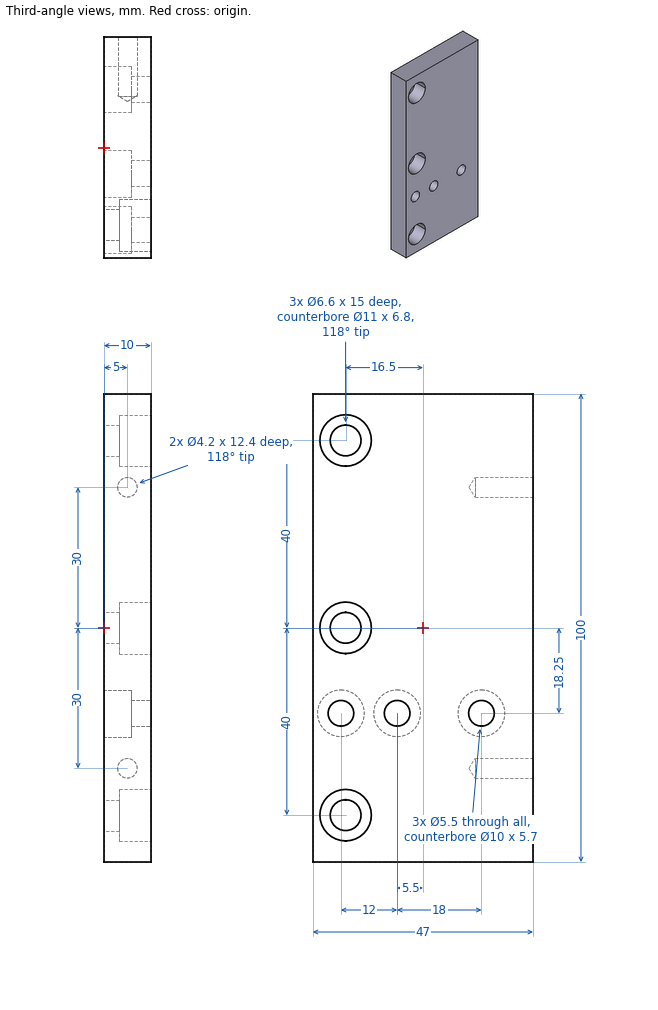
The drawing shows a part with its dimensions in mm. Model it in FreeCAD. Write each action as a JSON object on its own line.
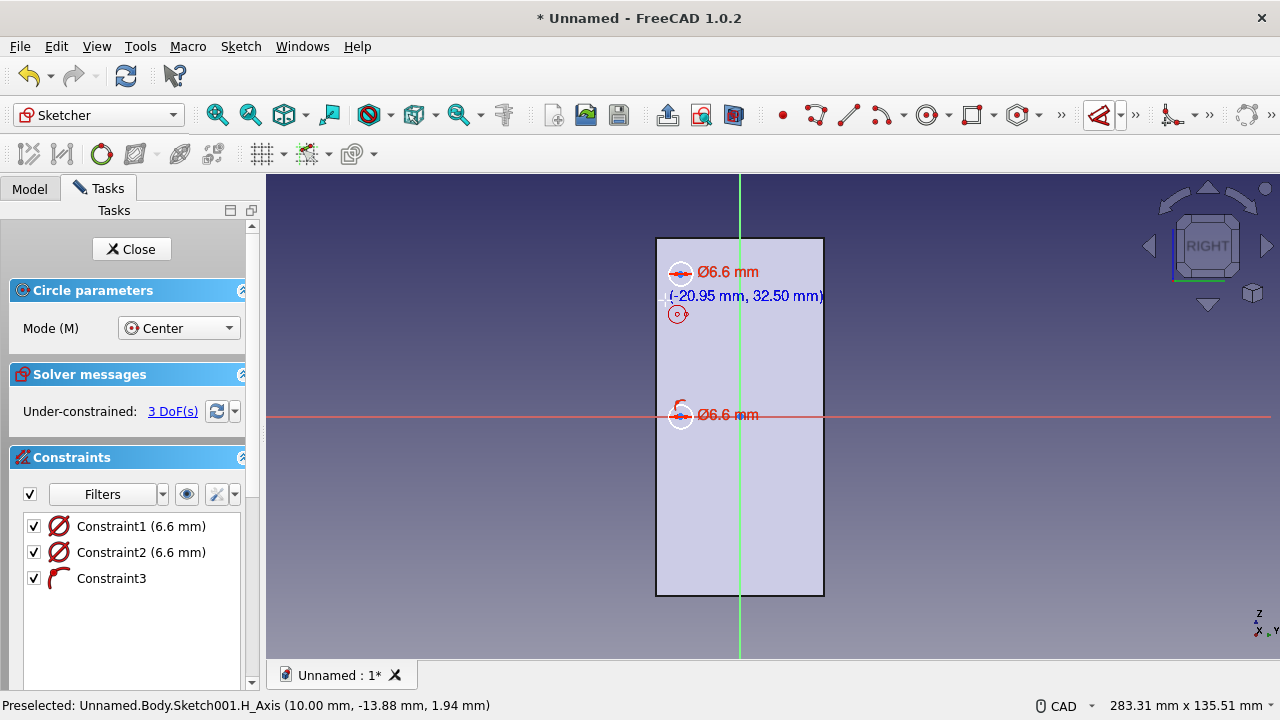
{"action": "scroll", "coordinate": [681, 560], "scroll_direction": "up", "scroll_amount": 4}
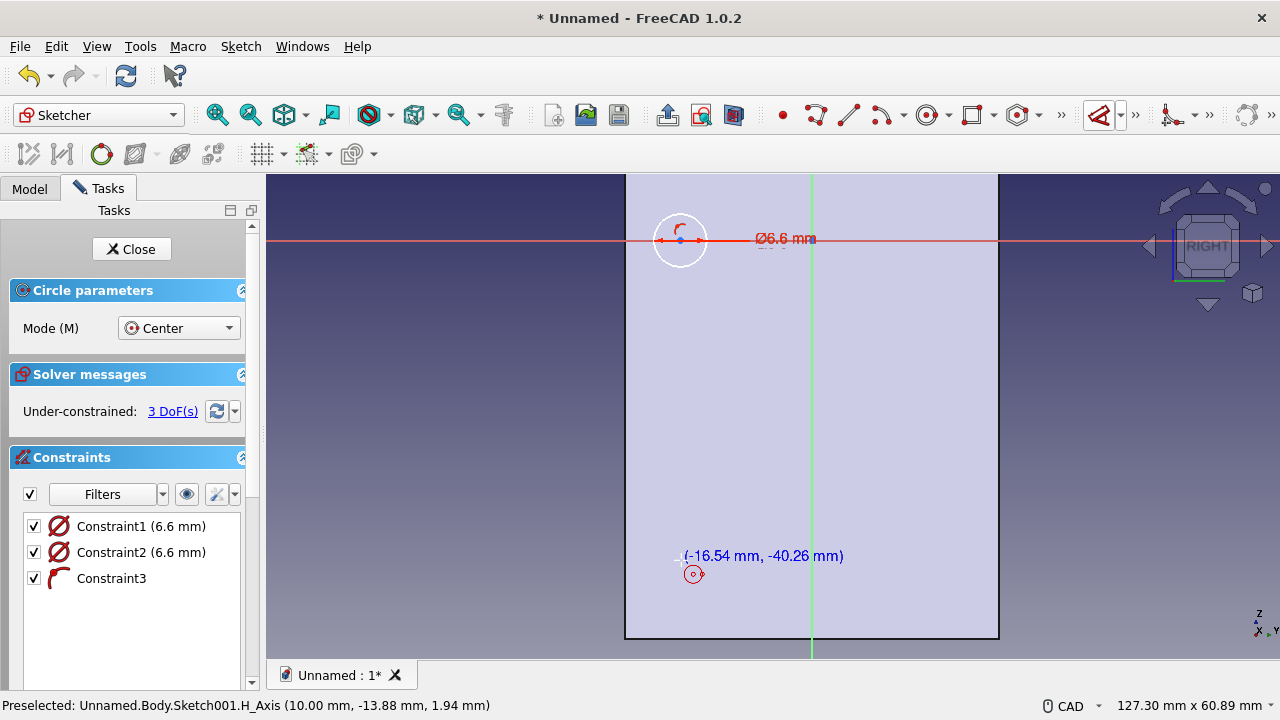
{"action": "left_click", "coordinate": [681, 559]}
{"action": "mouse_move", "coordinate": [699, 541]}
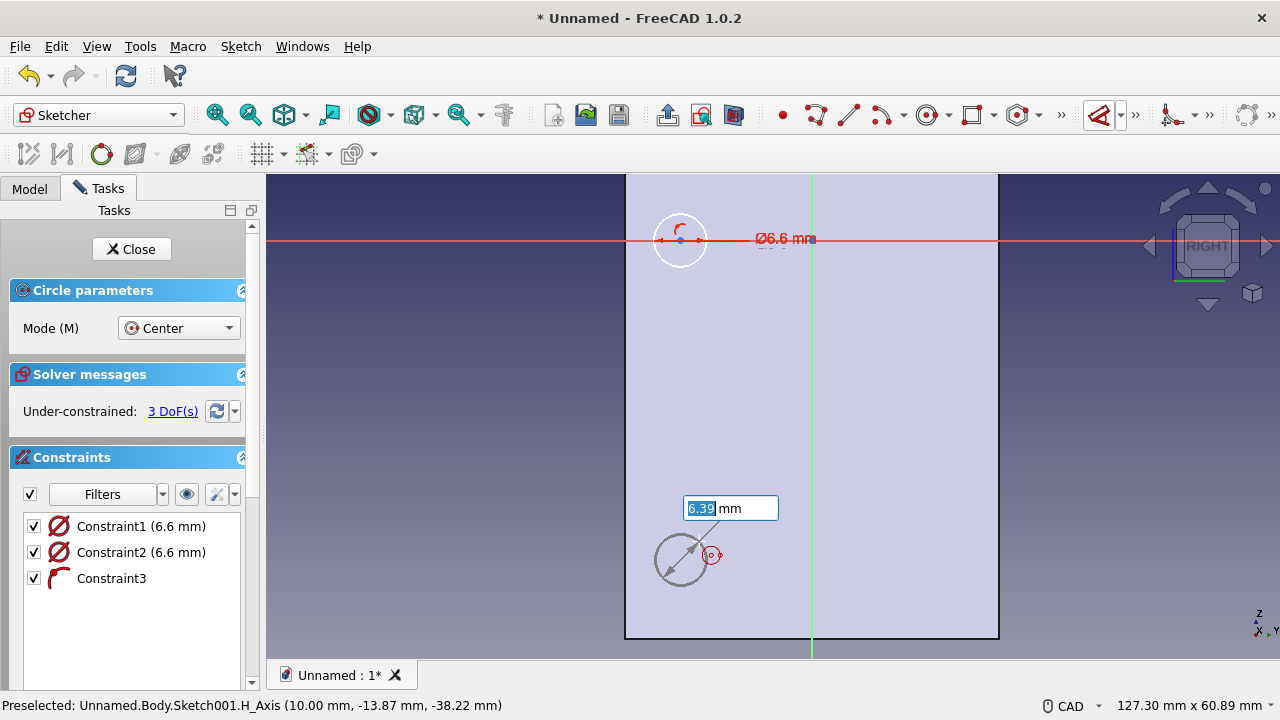
{"action": "type", "text": "6.6"}
{"action": "key", "text": "Return"}
{"action": "key", "text": "Escape"}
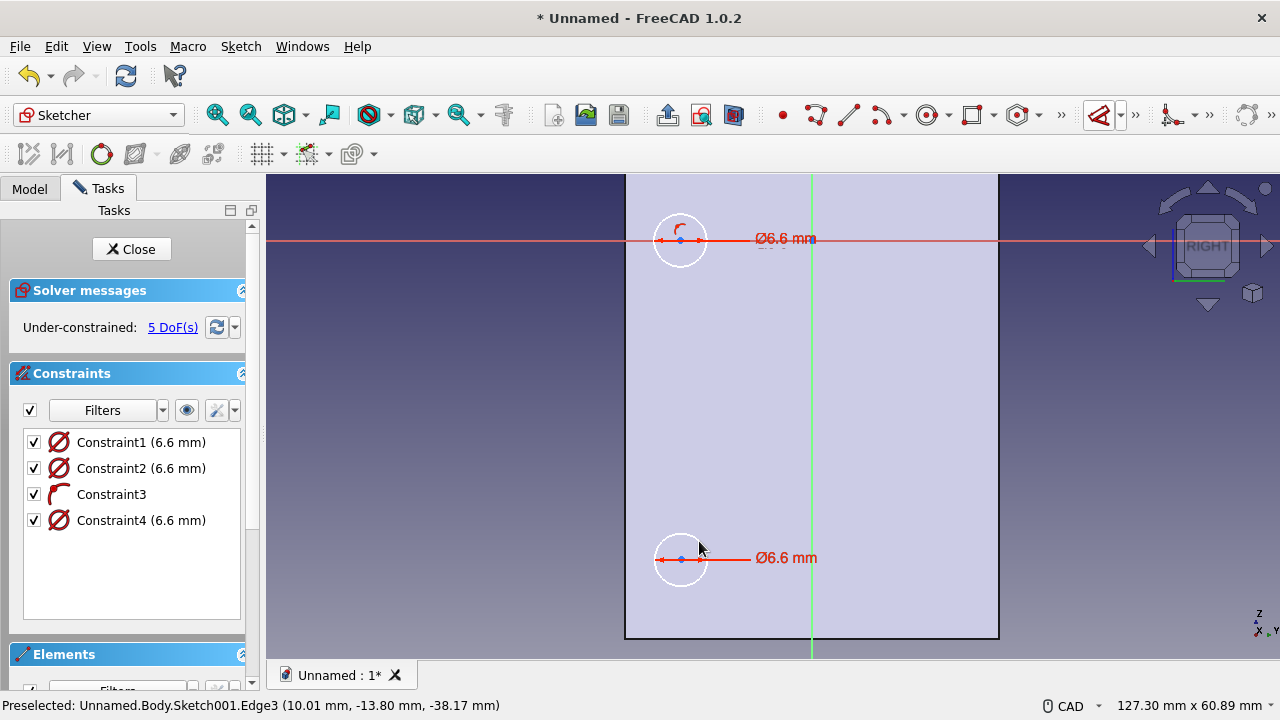
{"action": "scroll", "coordinate": [681, 560], "scroll_direction": "down", "scroll_amount": 4}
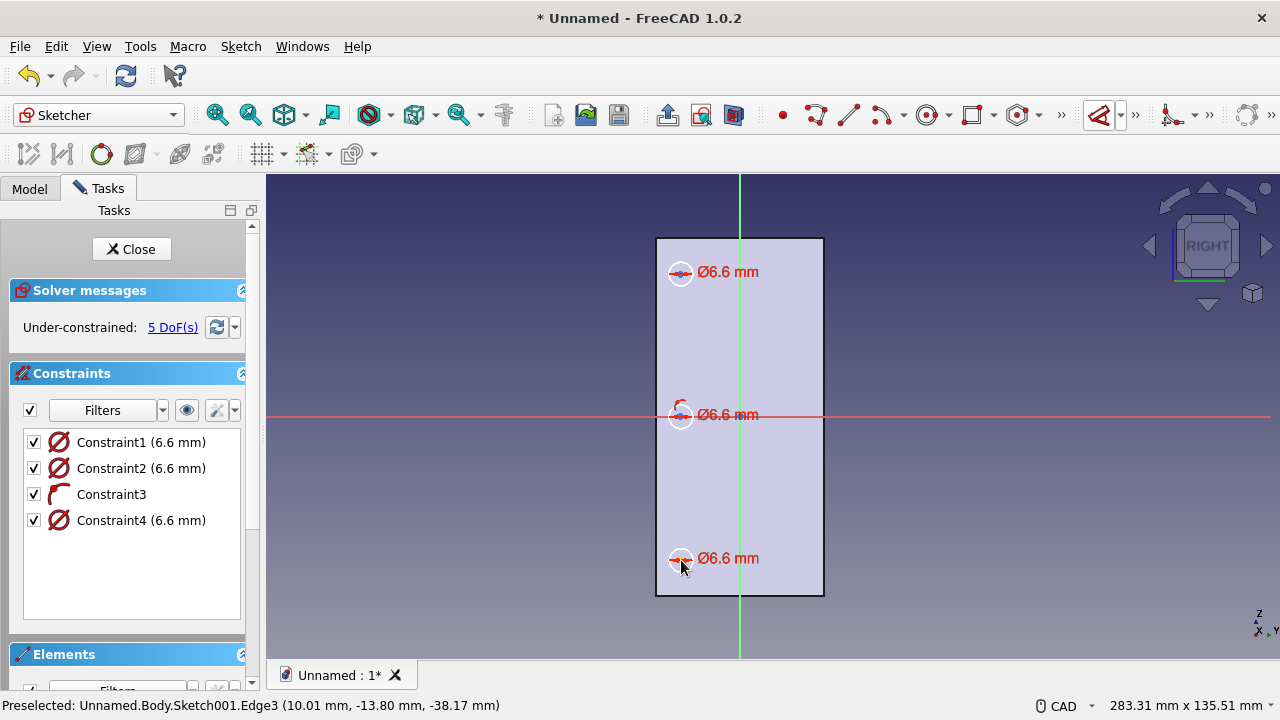
{"action": "left_click", "coordinate": [681, 274]}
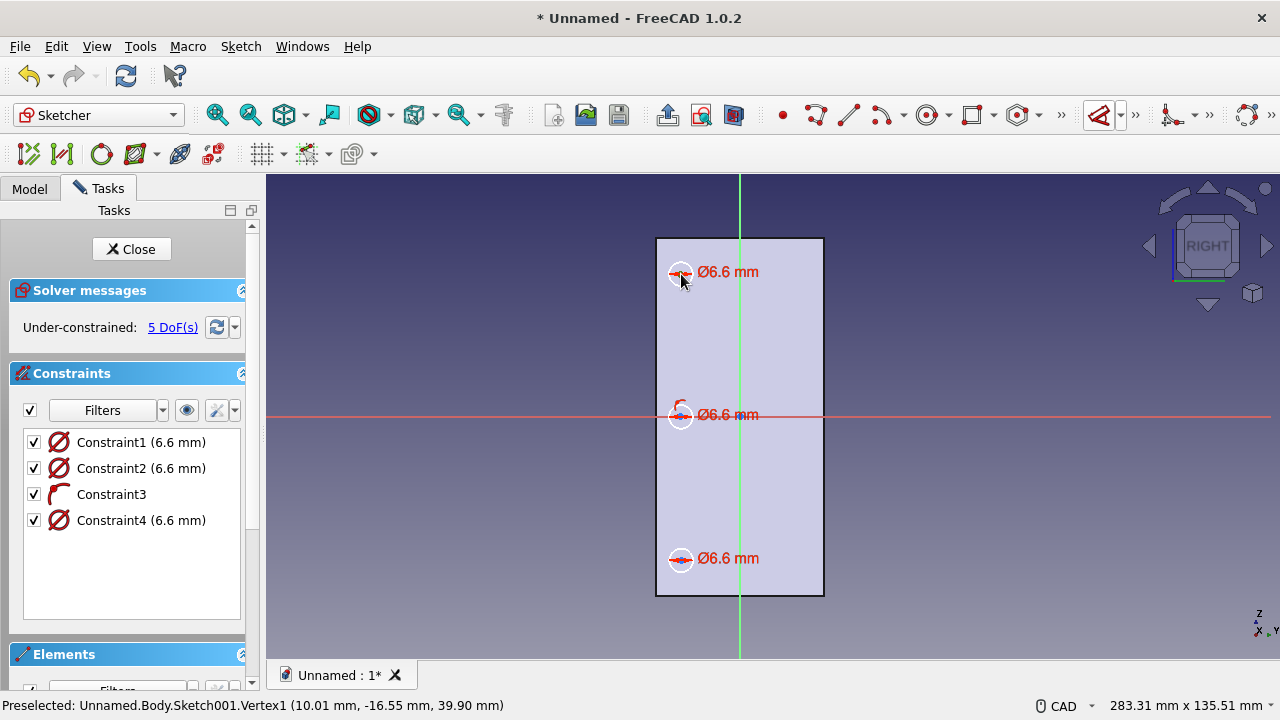
{"action": "left_click", "coordinate": [681, 417]}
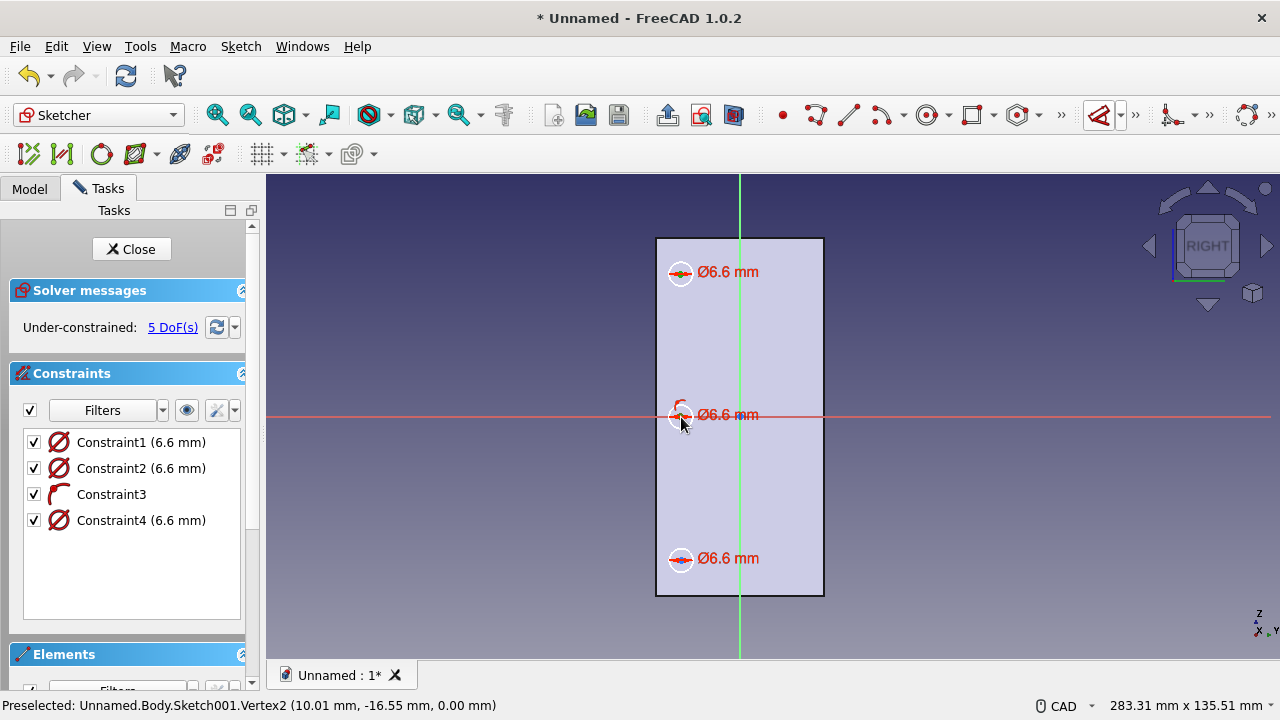
{"action": "key", "text": "v"}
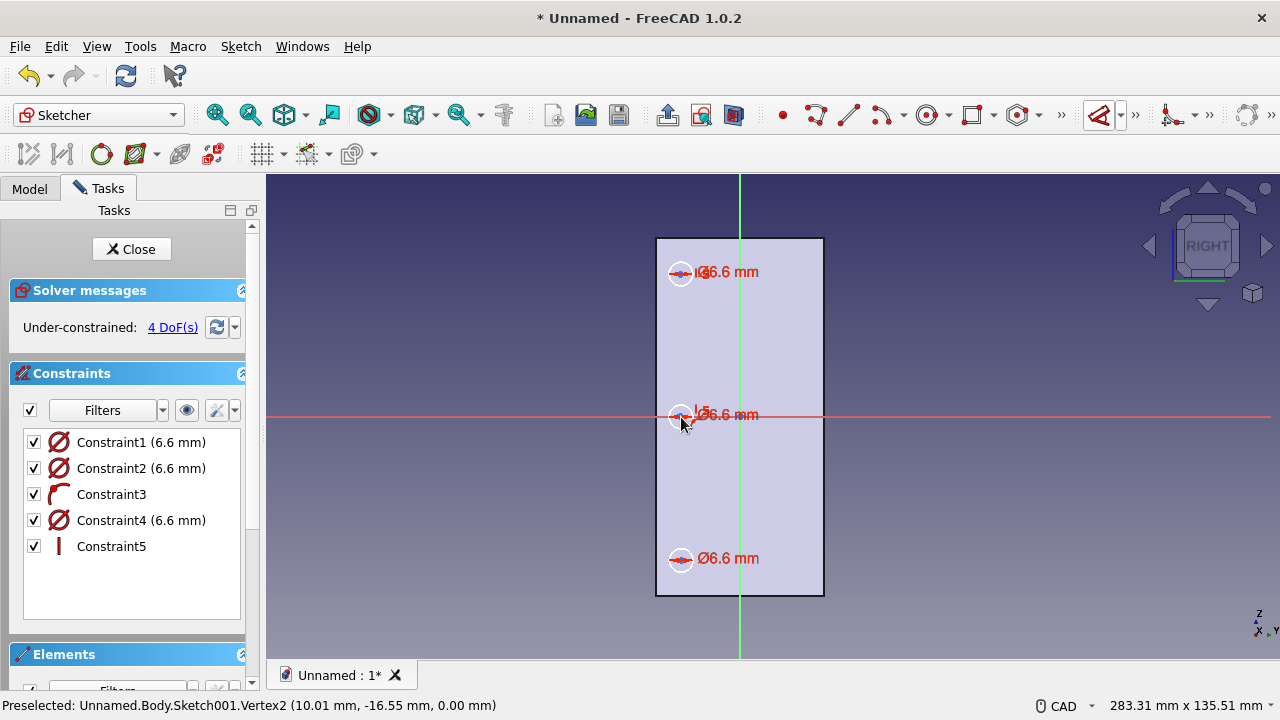
{"action": "left_click", "coordinate": [681, 417]}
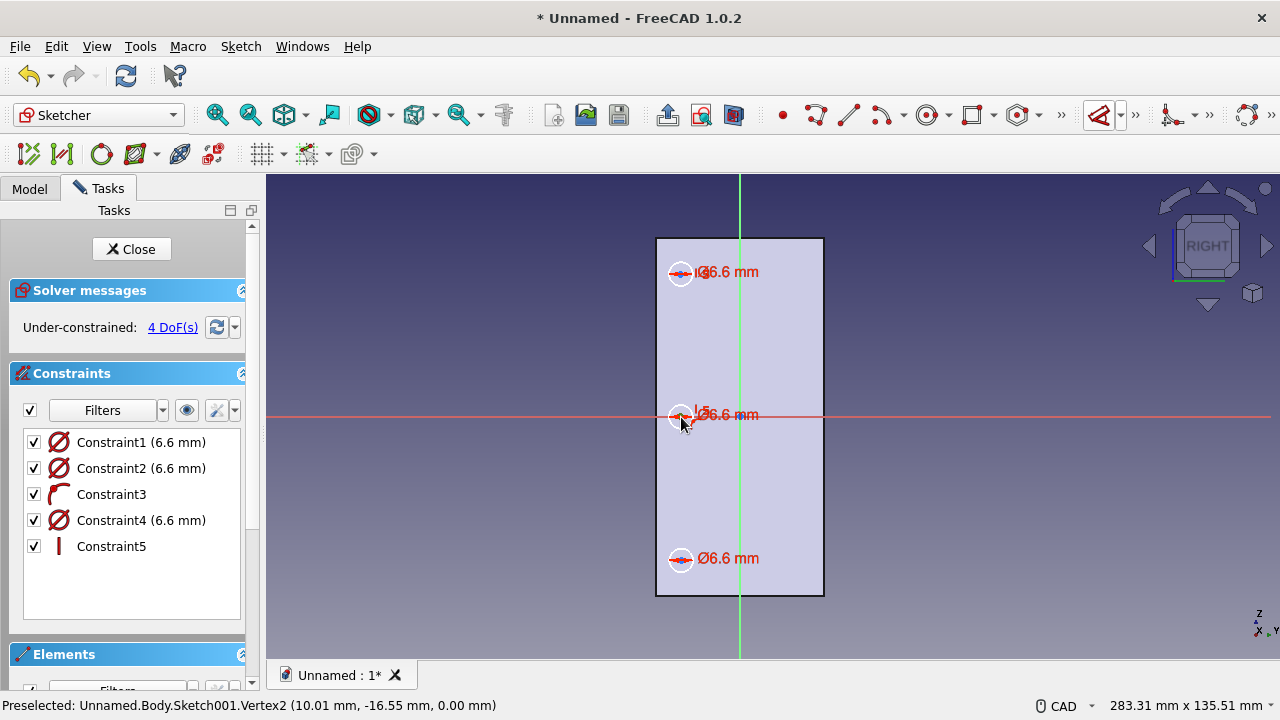
{"action": "left_click", "coordinate": [681, 560]}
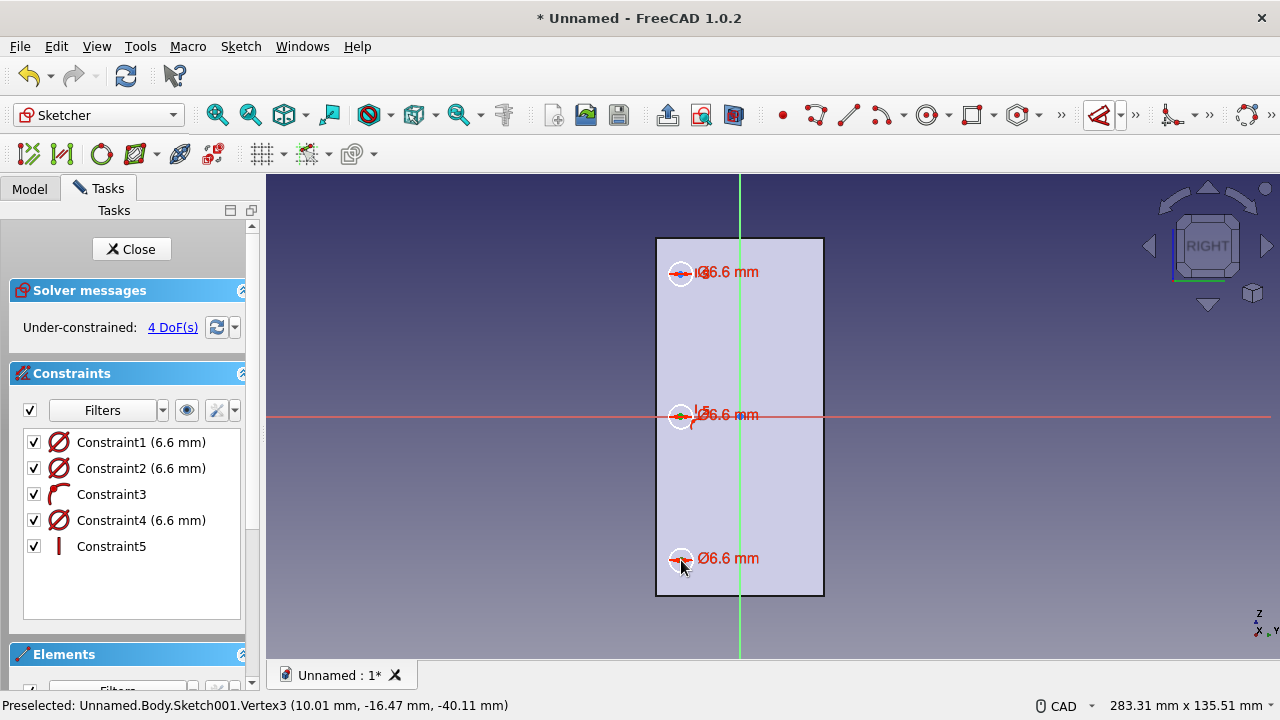
{"action": "key", "text": "v"}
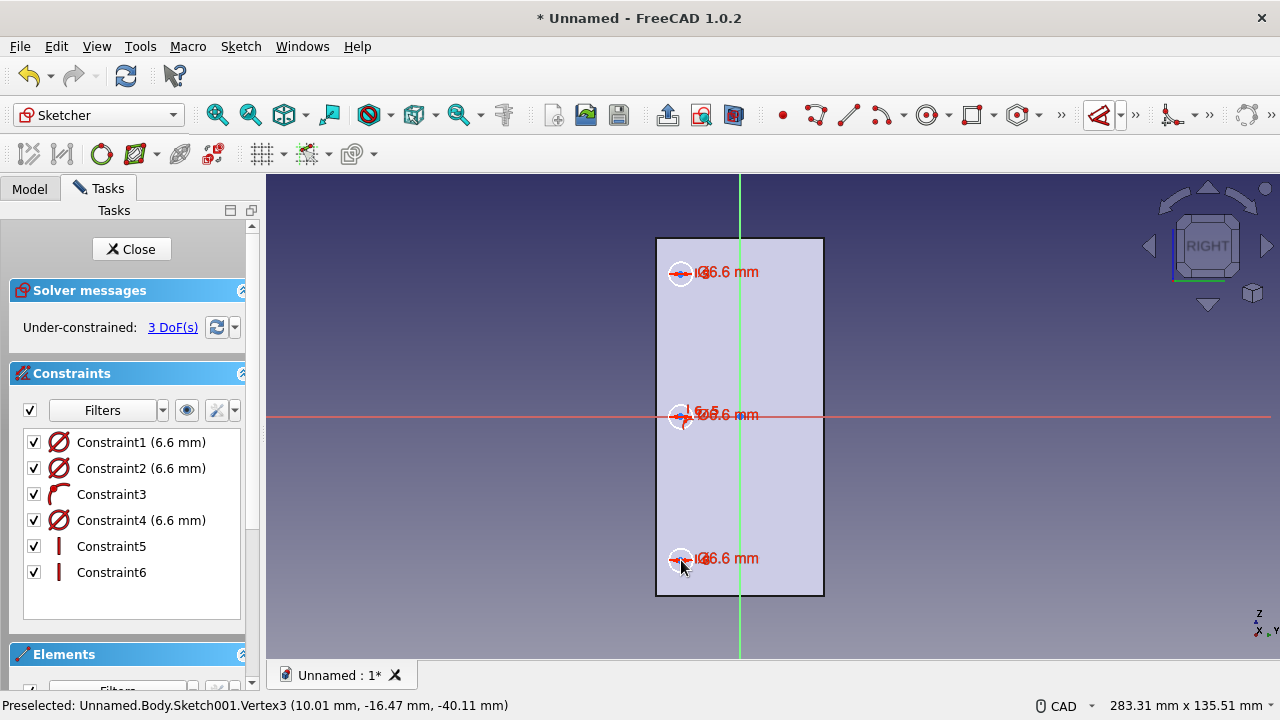
{"action": "left_click", "coordinate": [1098, 116]}